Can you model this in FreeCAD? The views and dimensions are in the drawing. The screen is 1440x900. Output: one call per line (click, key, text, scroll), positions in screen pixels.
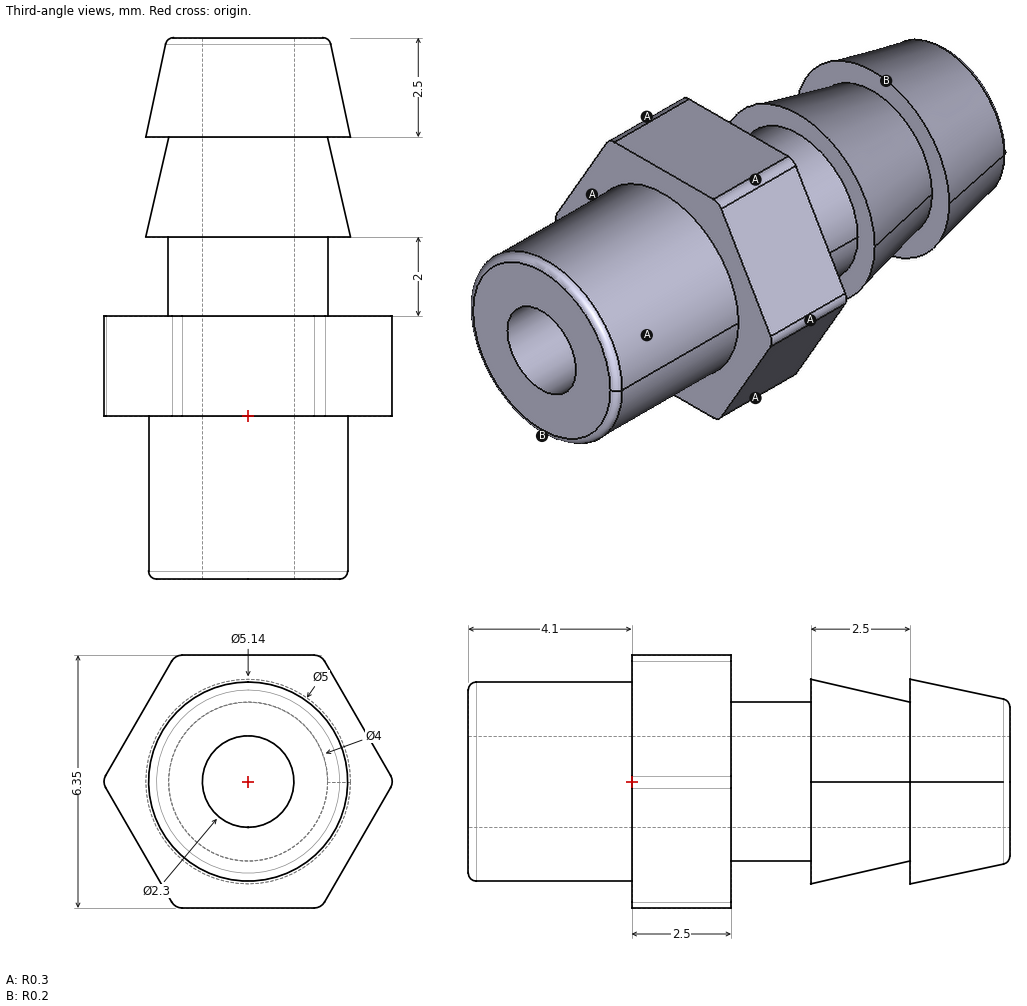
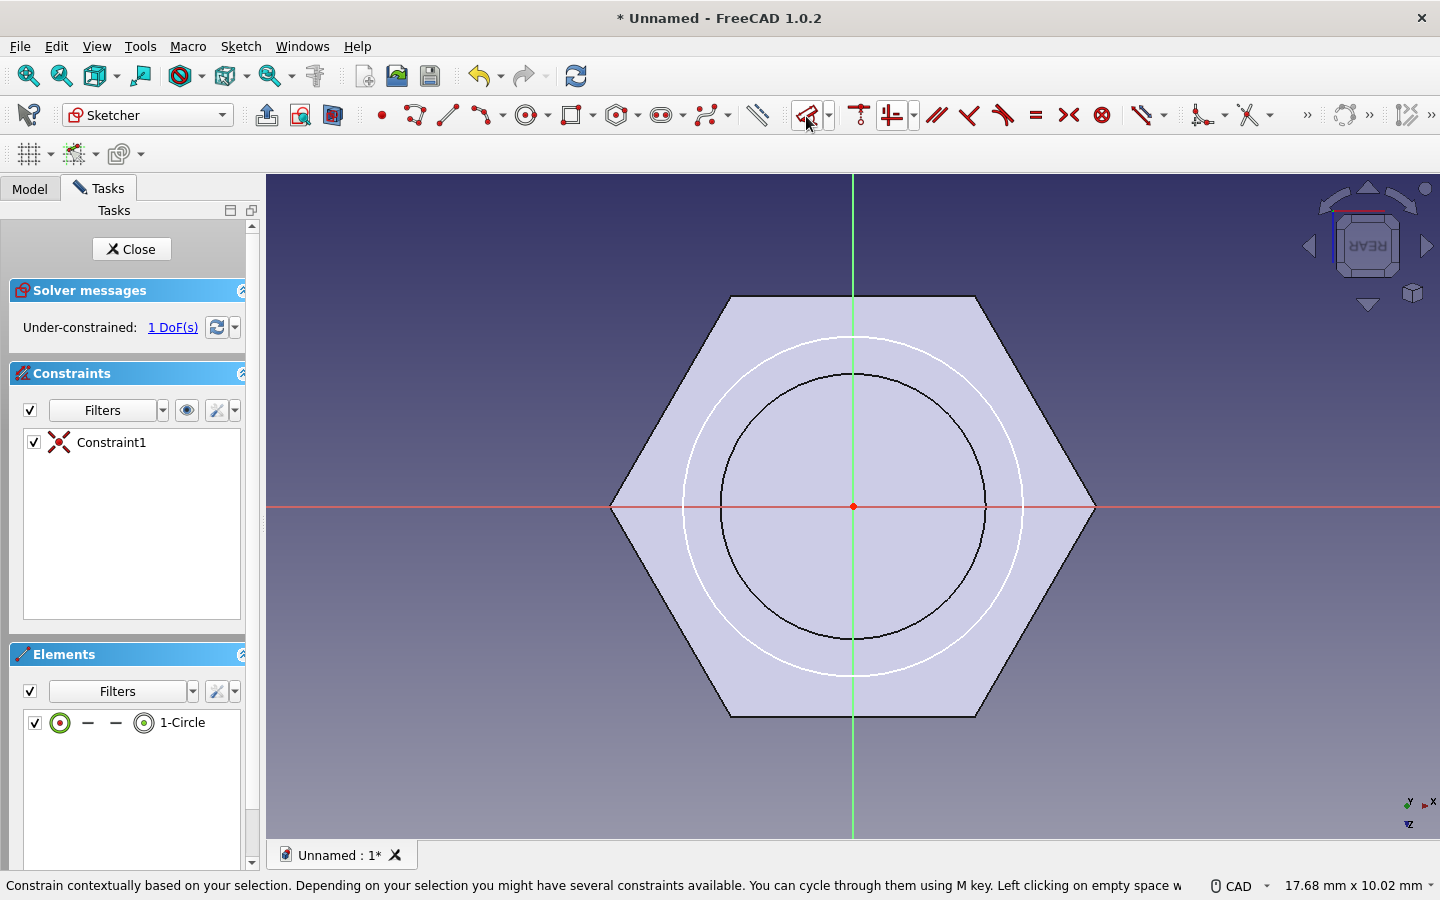
click(973, 386)
click(996, 363)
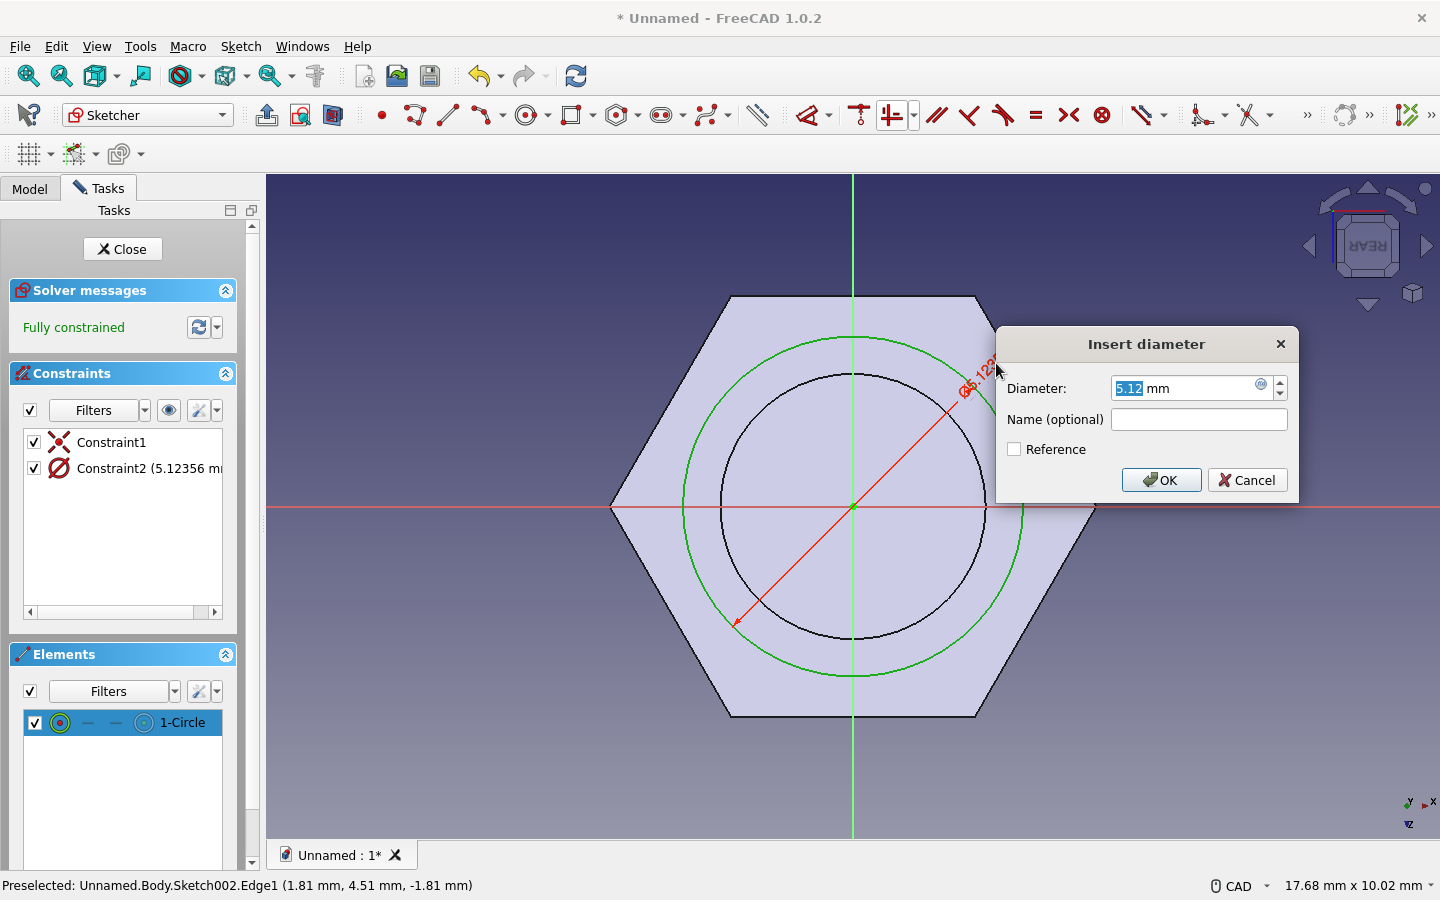
text(5.14)
key(Return)
key(Escape)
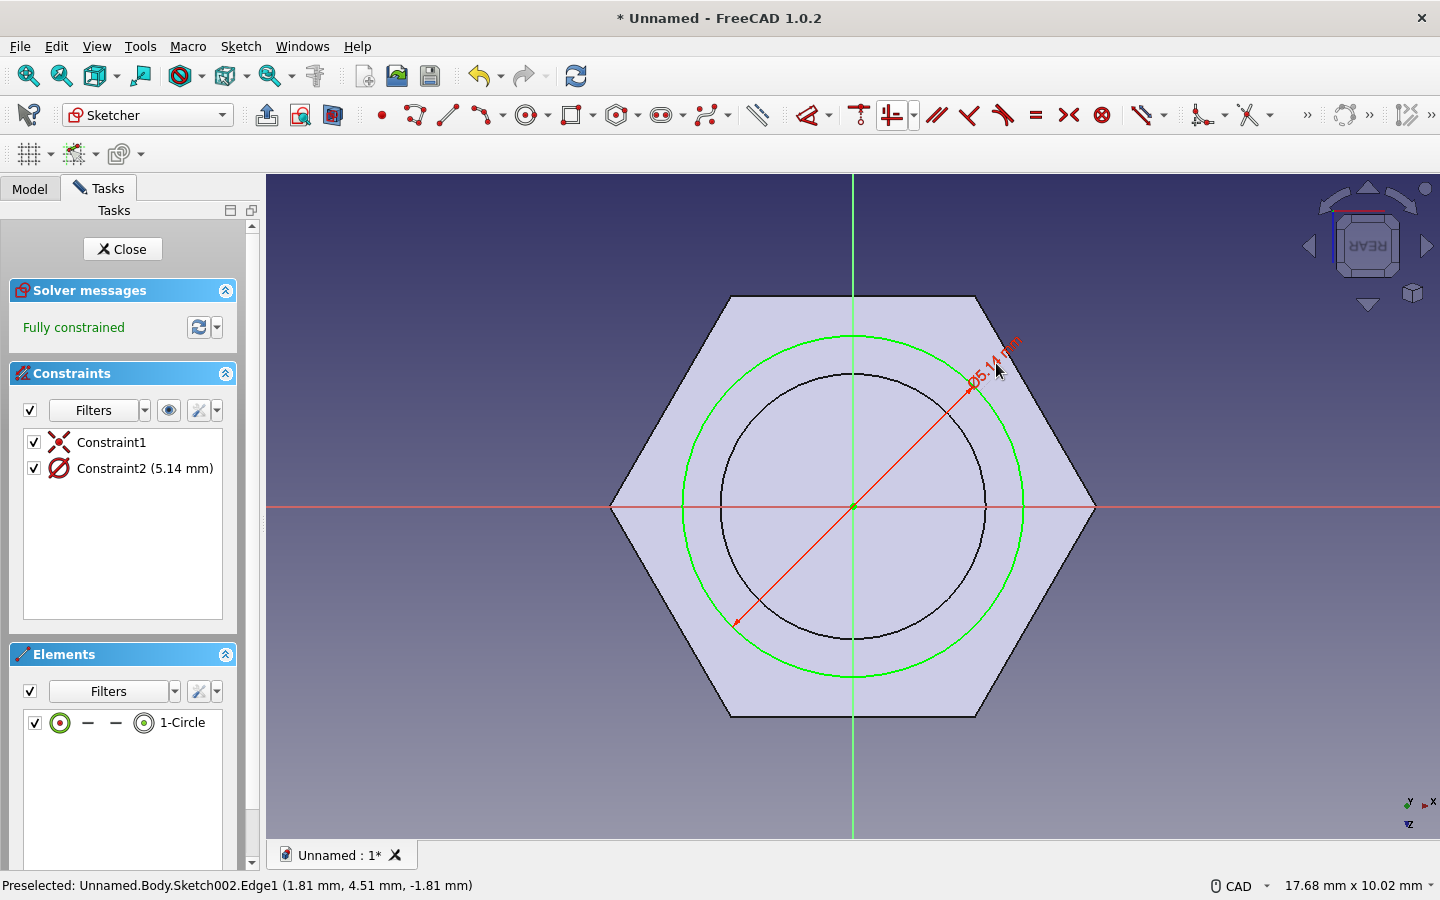
click(123, 249)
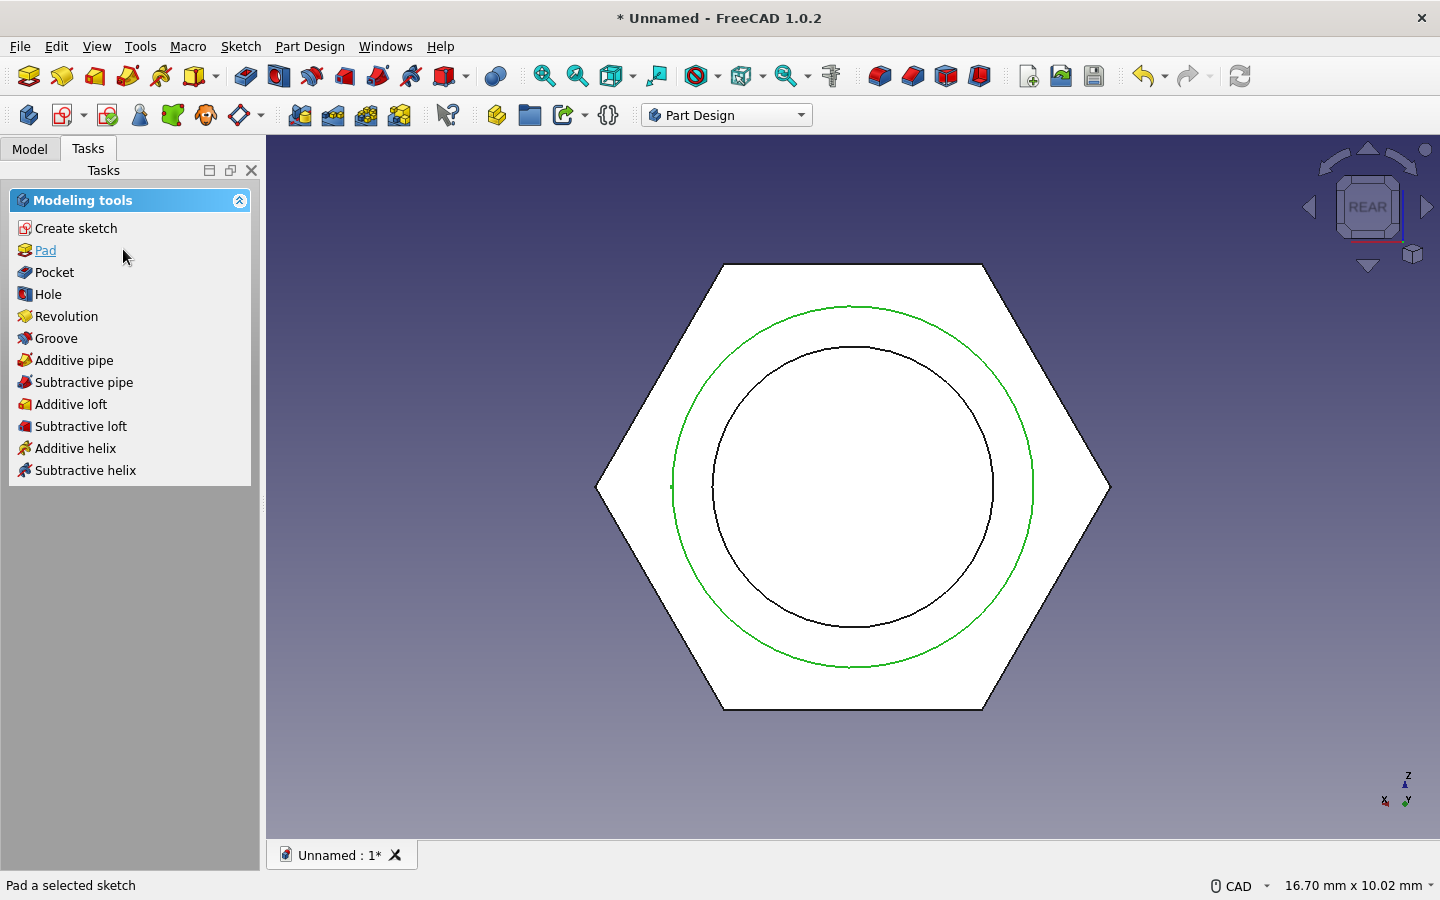
click(29, 76)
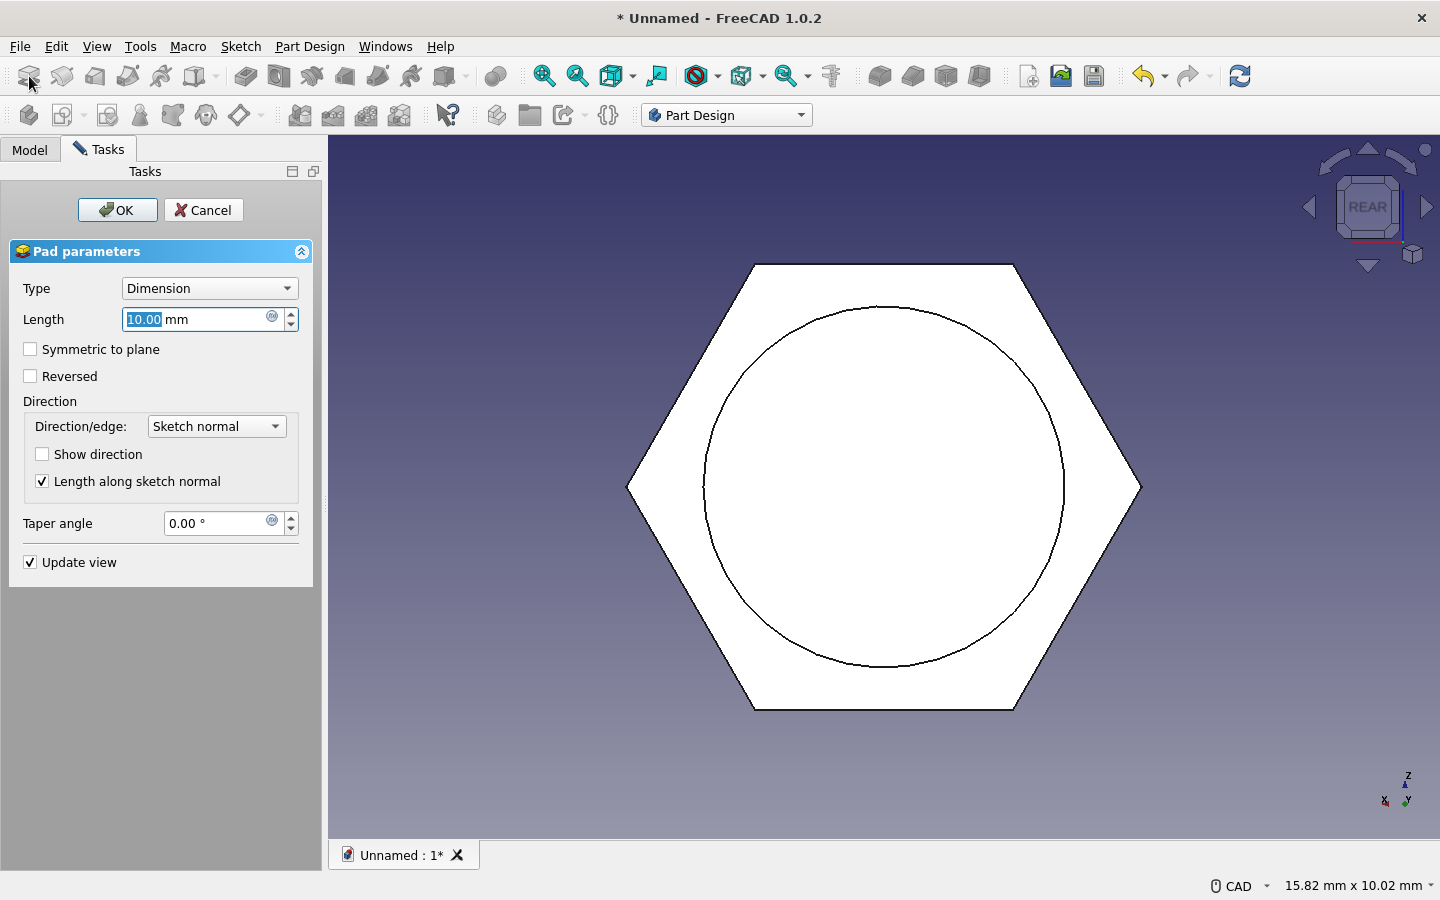
text(2.5)
key(Tab)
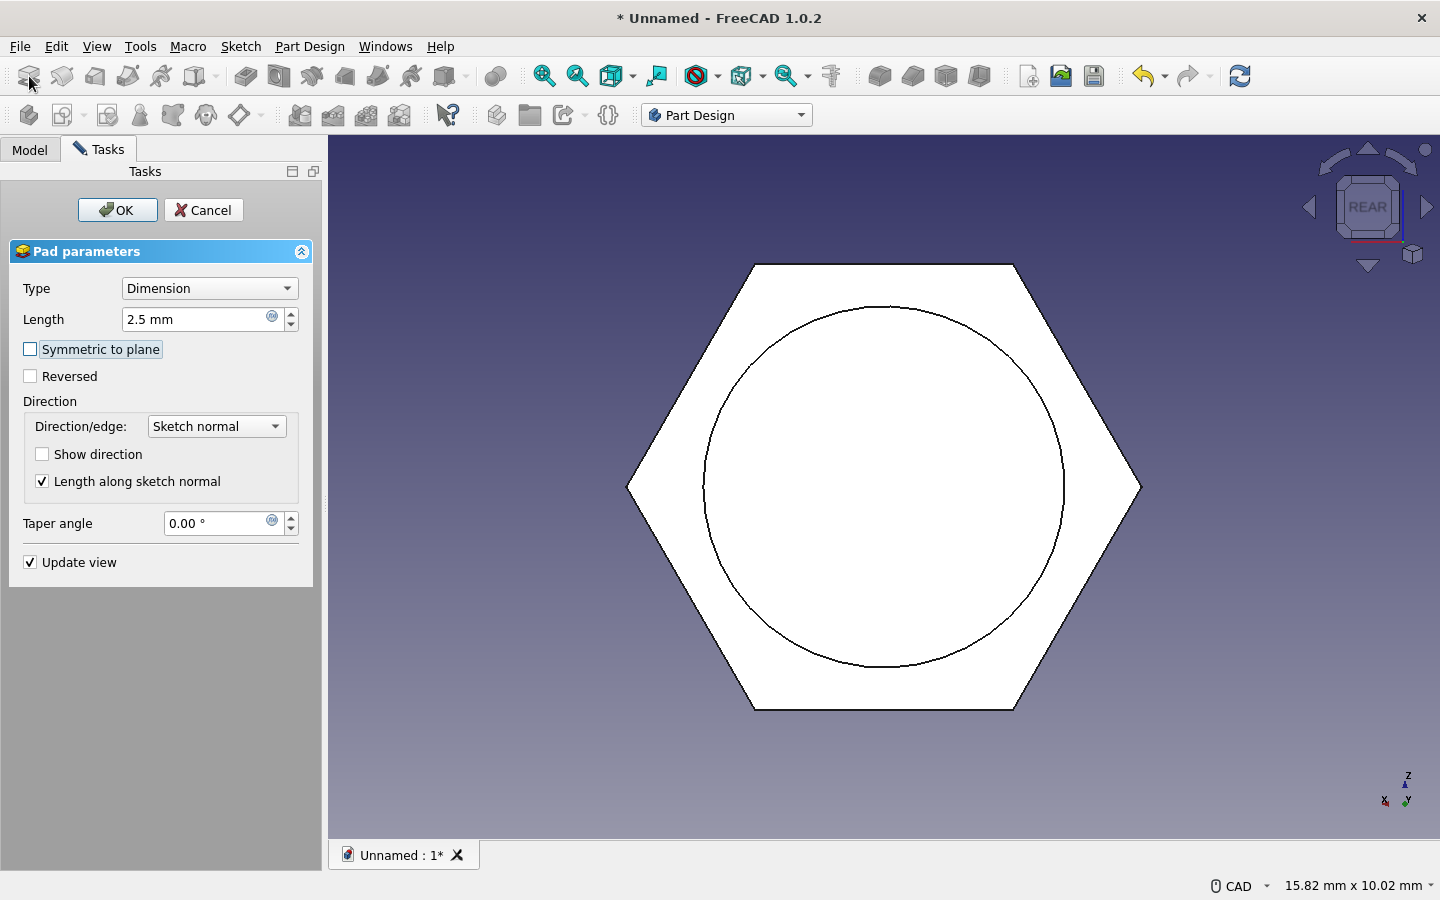
triple_click(224, 524)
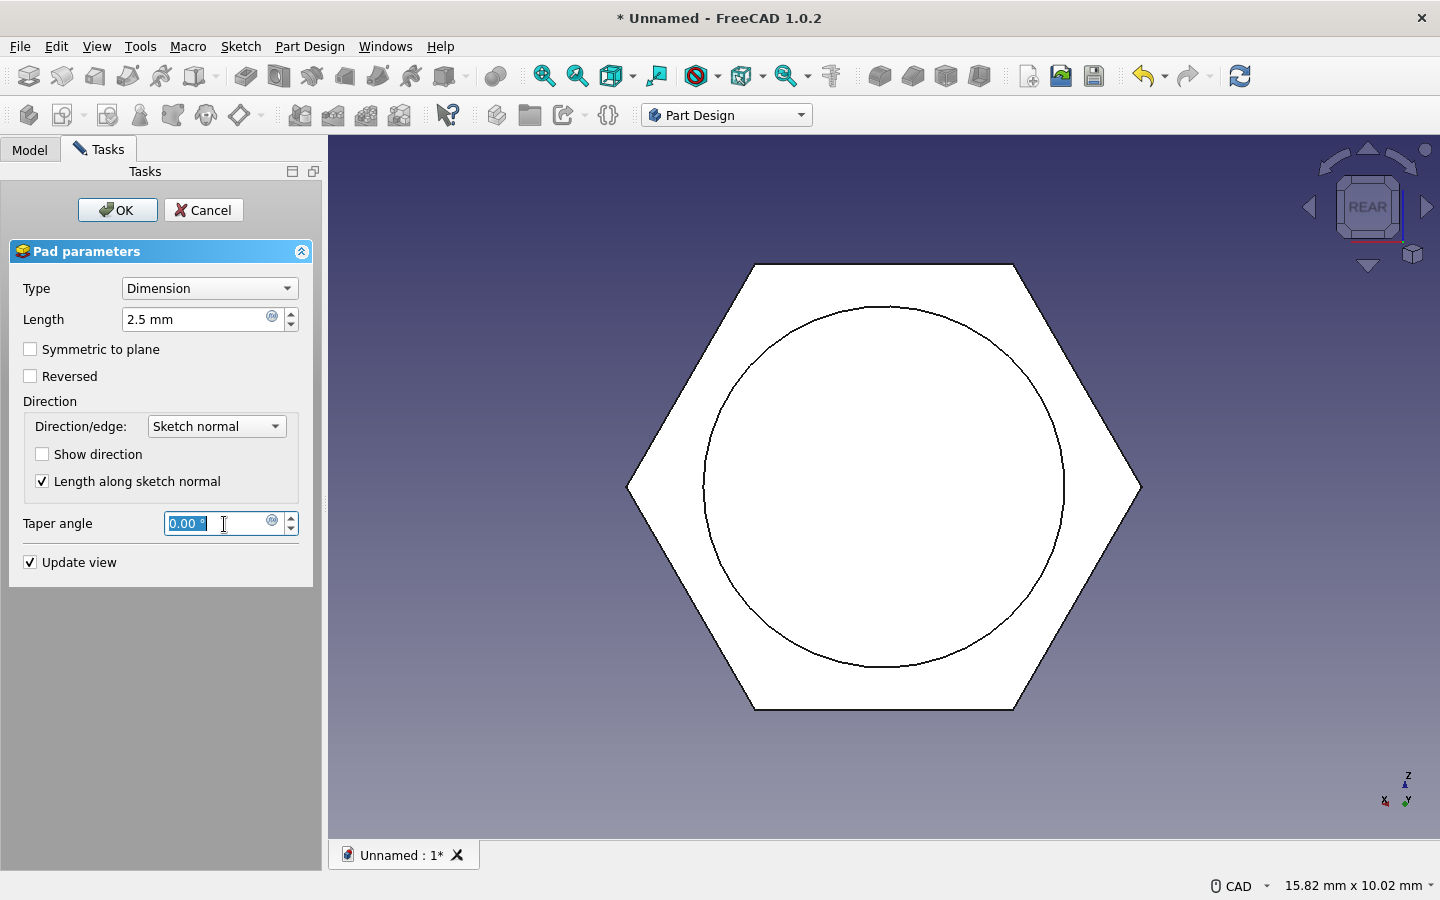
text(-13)
key(Tab)